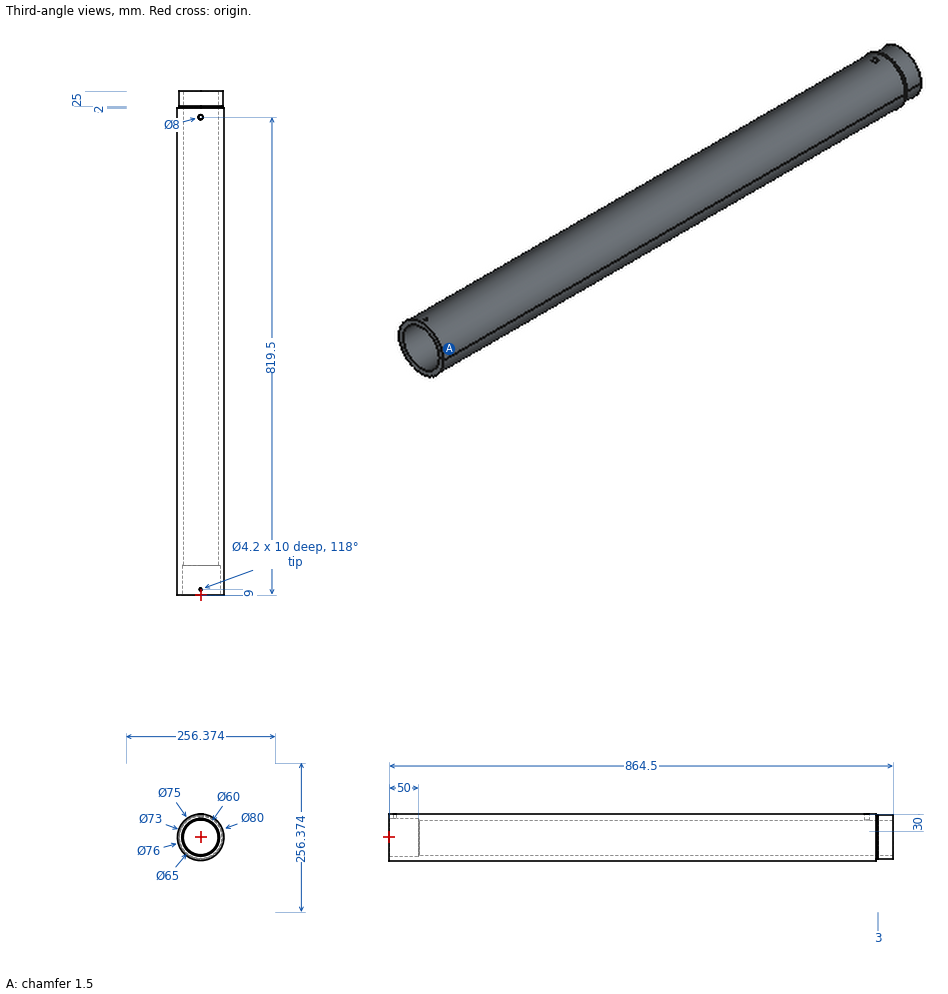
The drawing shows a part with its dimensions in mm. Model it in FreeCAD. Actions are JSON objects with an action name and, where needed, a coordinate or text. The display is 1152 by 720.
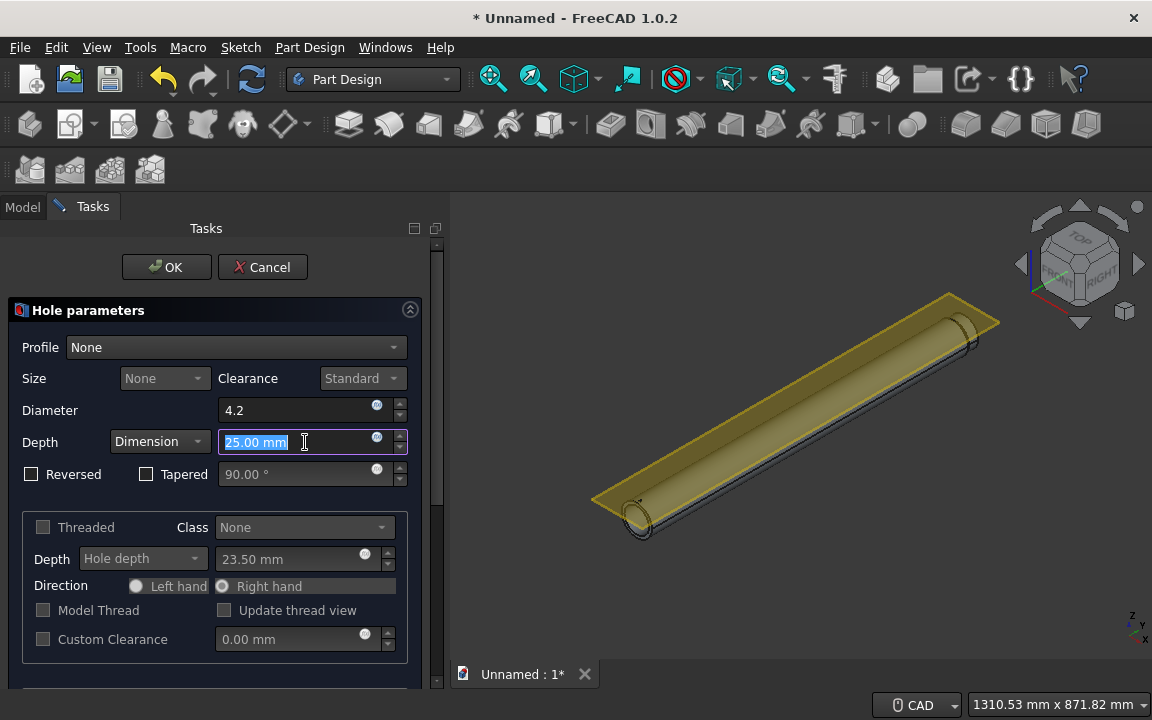
{"action": "type", "text": "10"}
{"action": "key", "text": "Tab"}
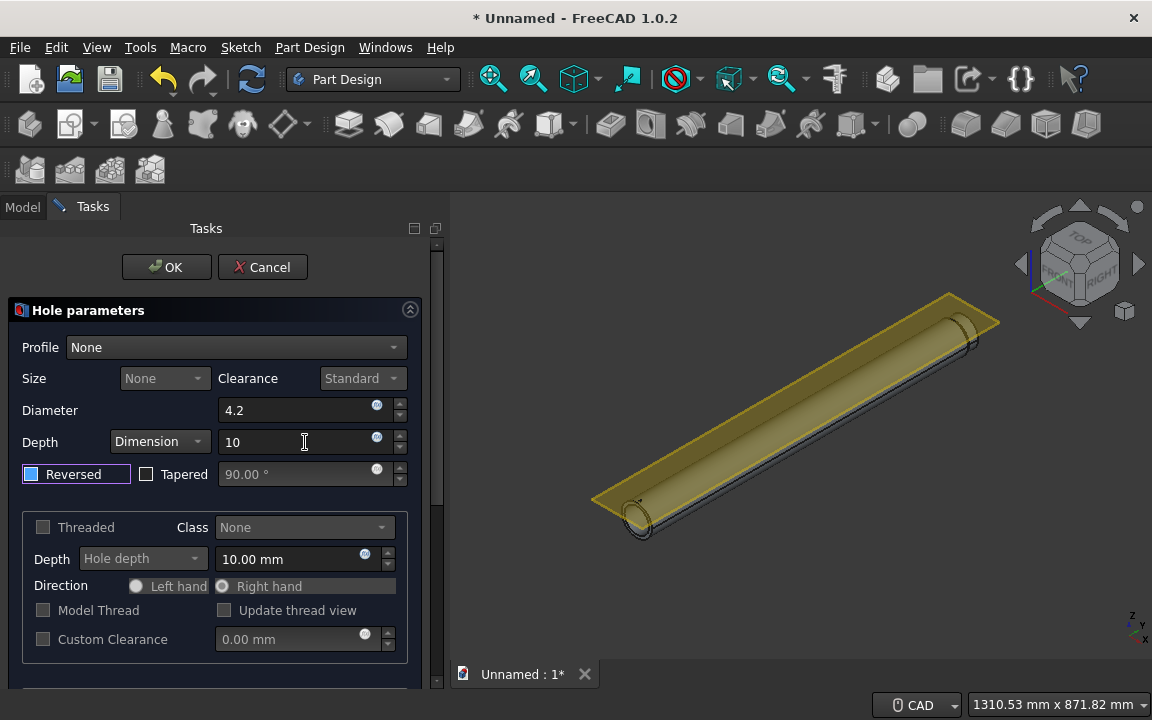
{"action": "left_click", "coordinate": [167, 267]}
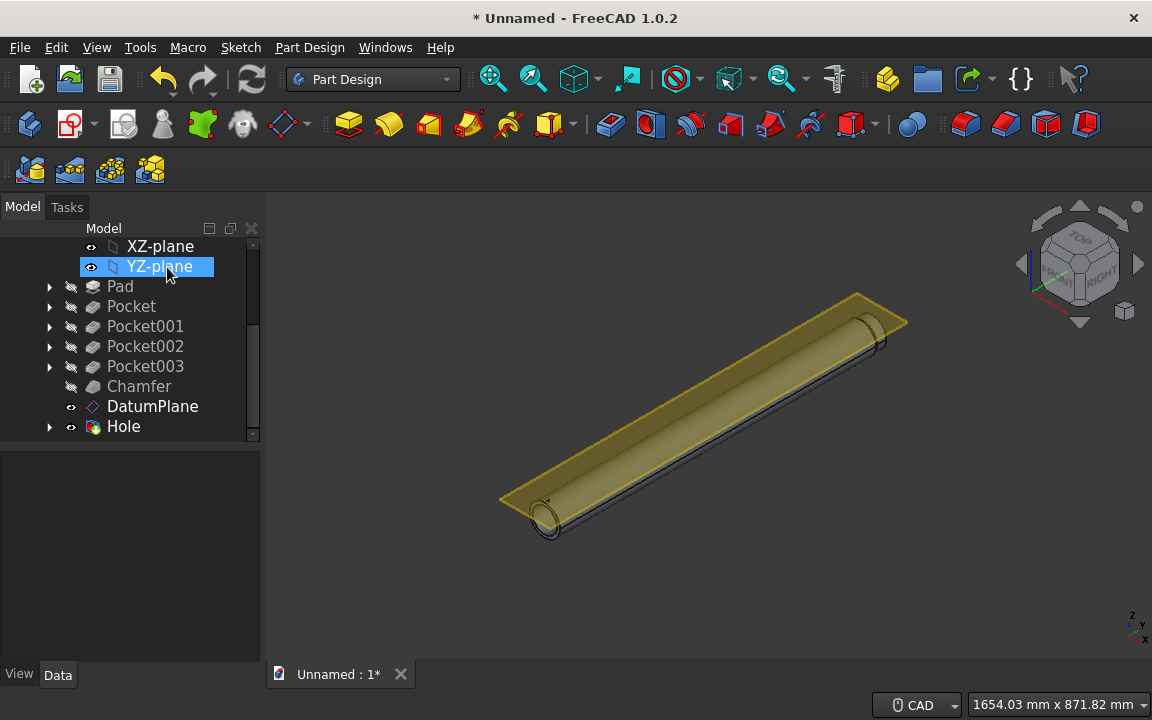
{"action": "left_click", "coordinate": [116, 407]}
{"action": "key", "text": "space"}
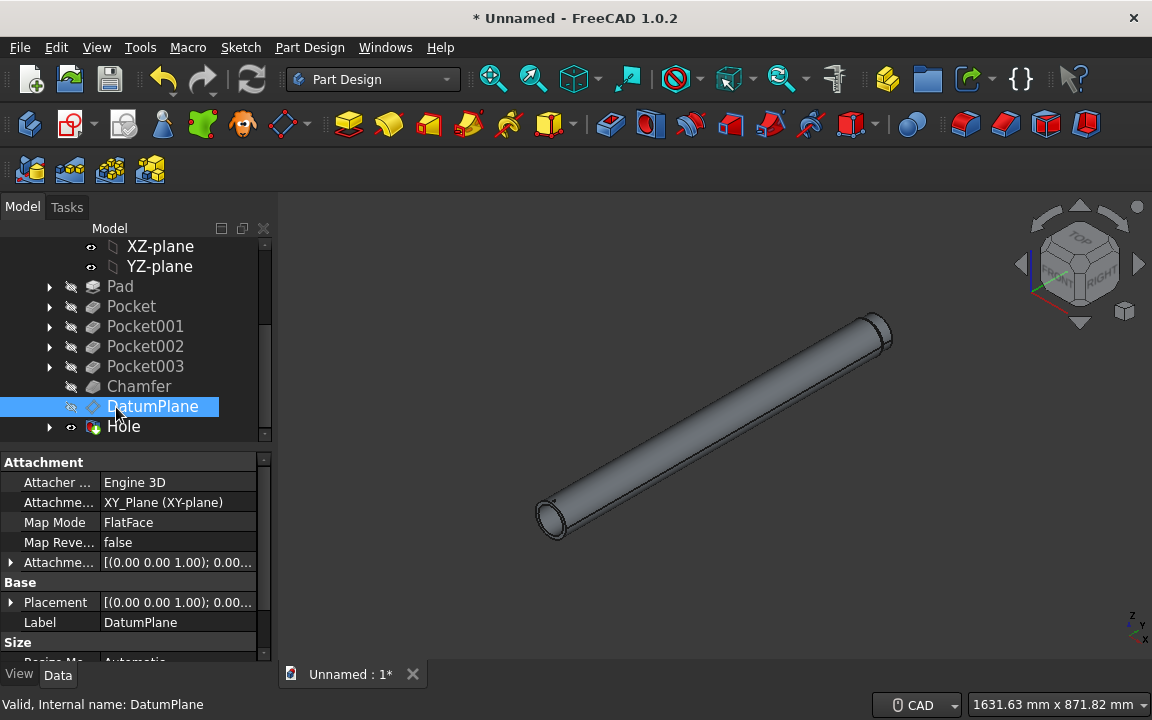
{"action": "scroll", "coordinate": [160, 342], "scroll_direction": "down", "scroll_amount": 3}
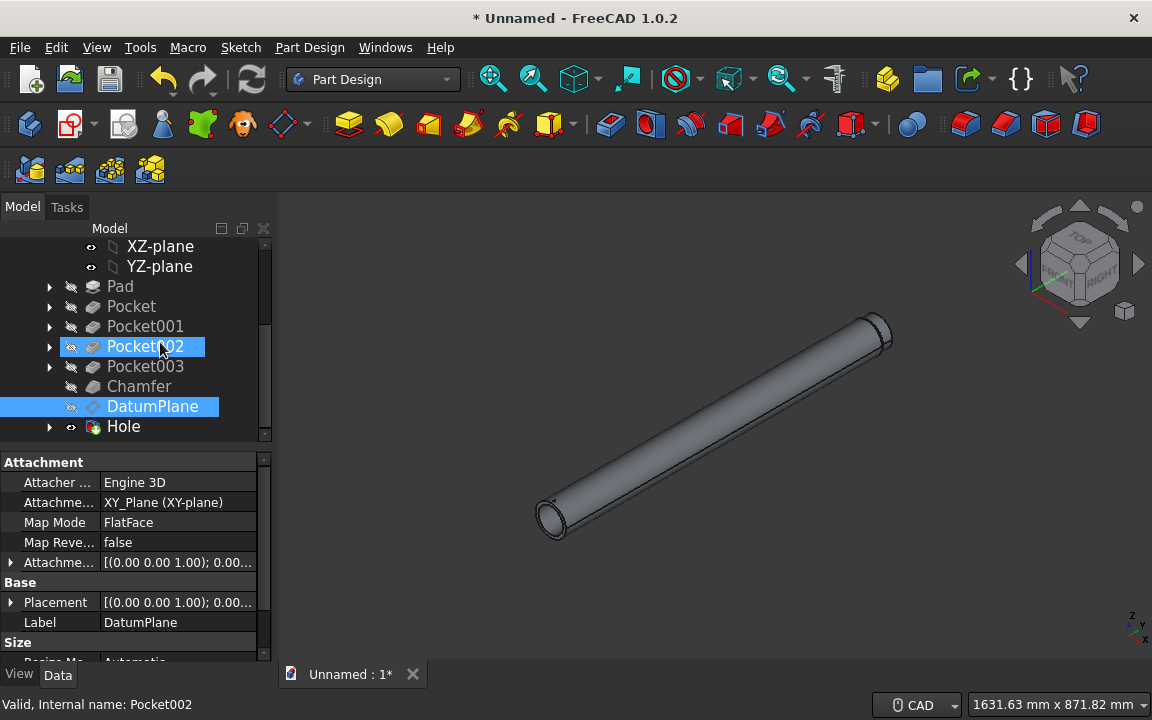
{"action": "scroll", "coordinate": [160, 342], "scroll_direction": "up", "scroll_amount": 15}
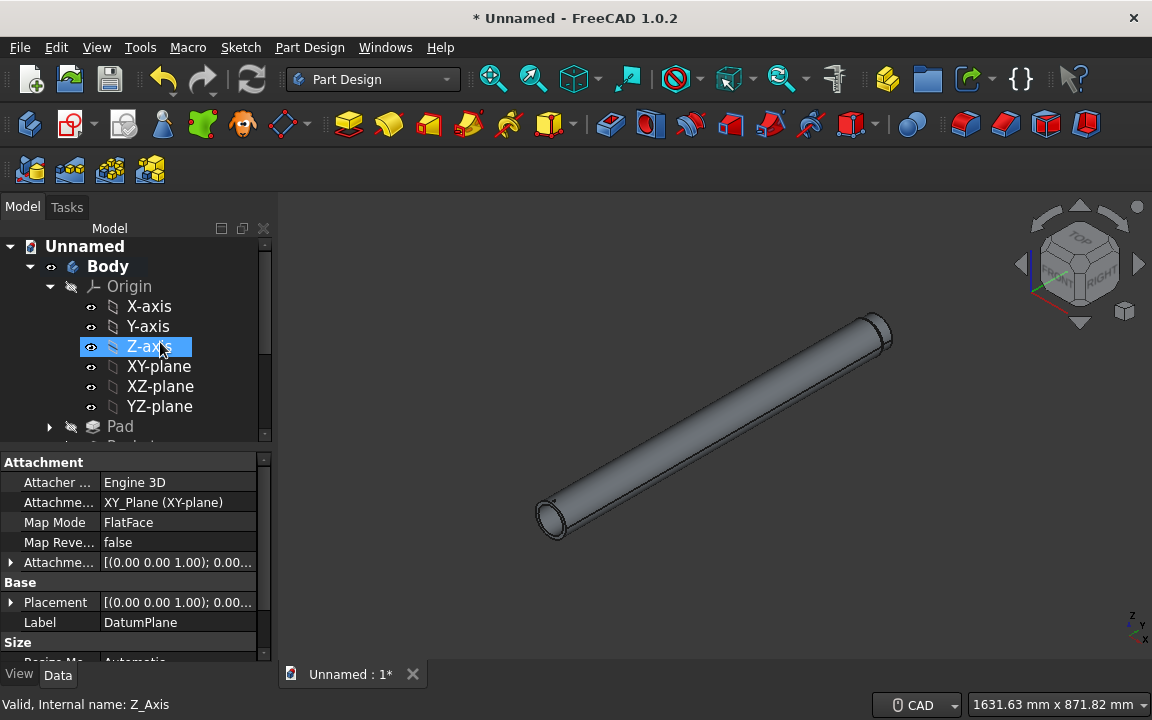
{"action": "left_click", "coordinate": [136, 367]}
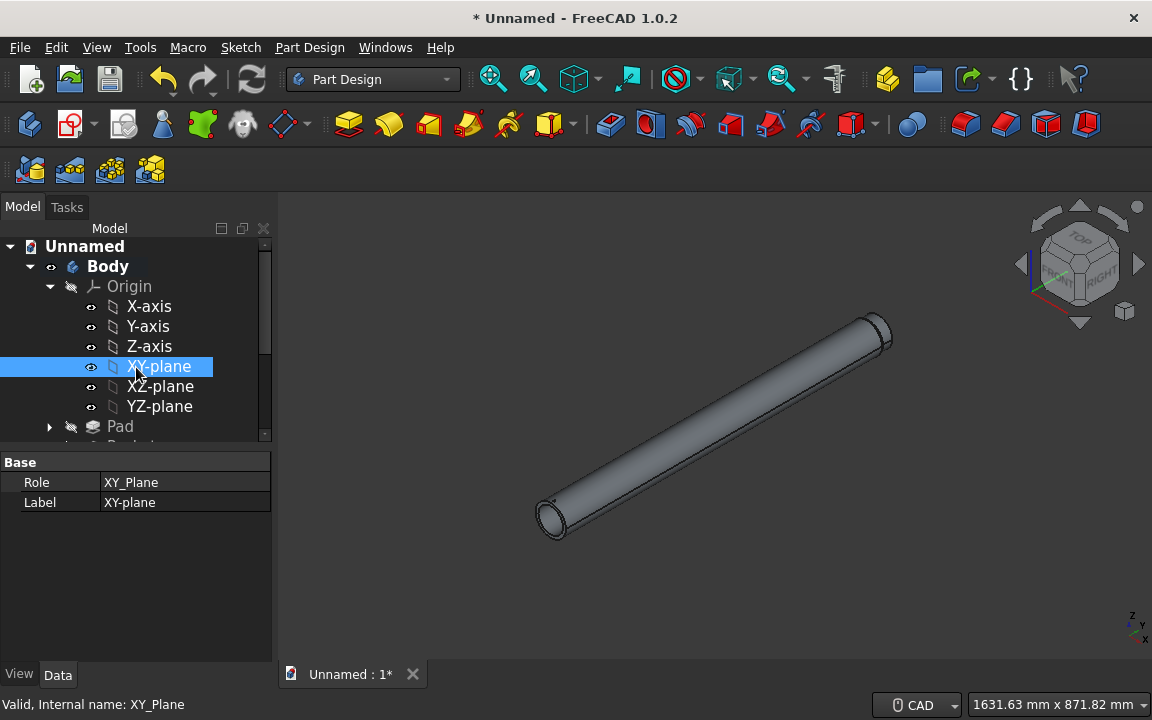
{"action": "left_click", "coordinate": [284, 124]}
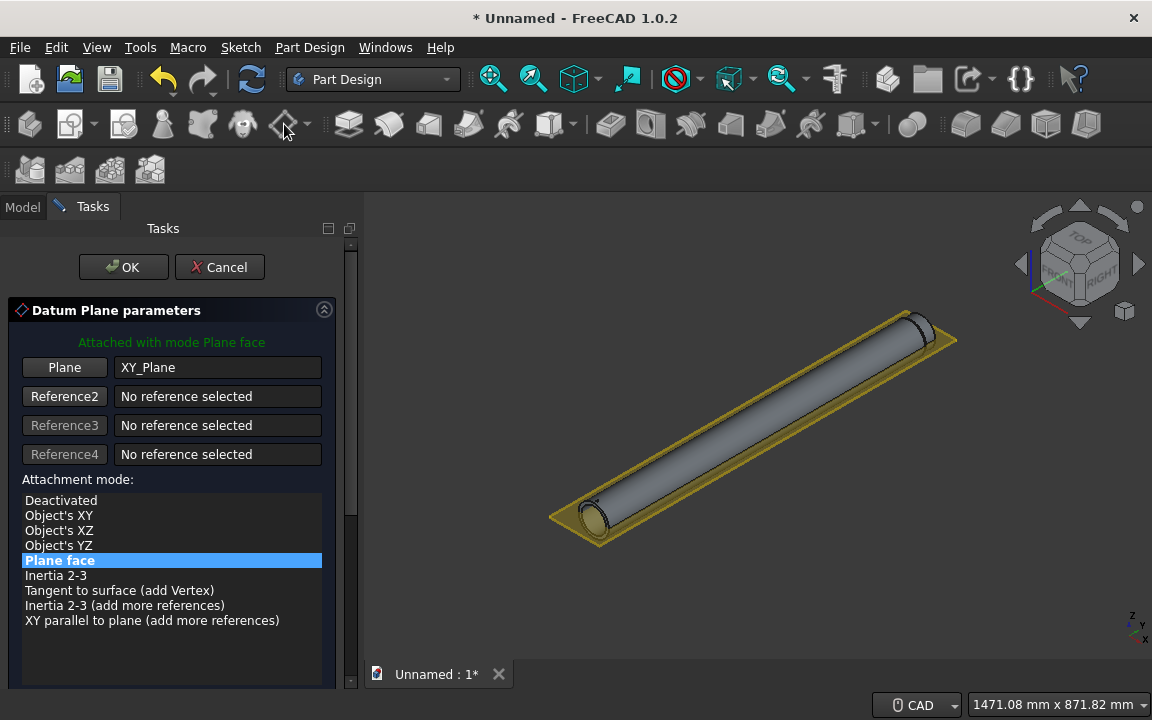
{"action": "scroll", "coordinate": [351, 463], "scroll_direction": "down", "scroll_amount": 3}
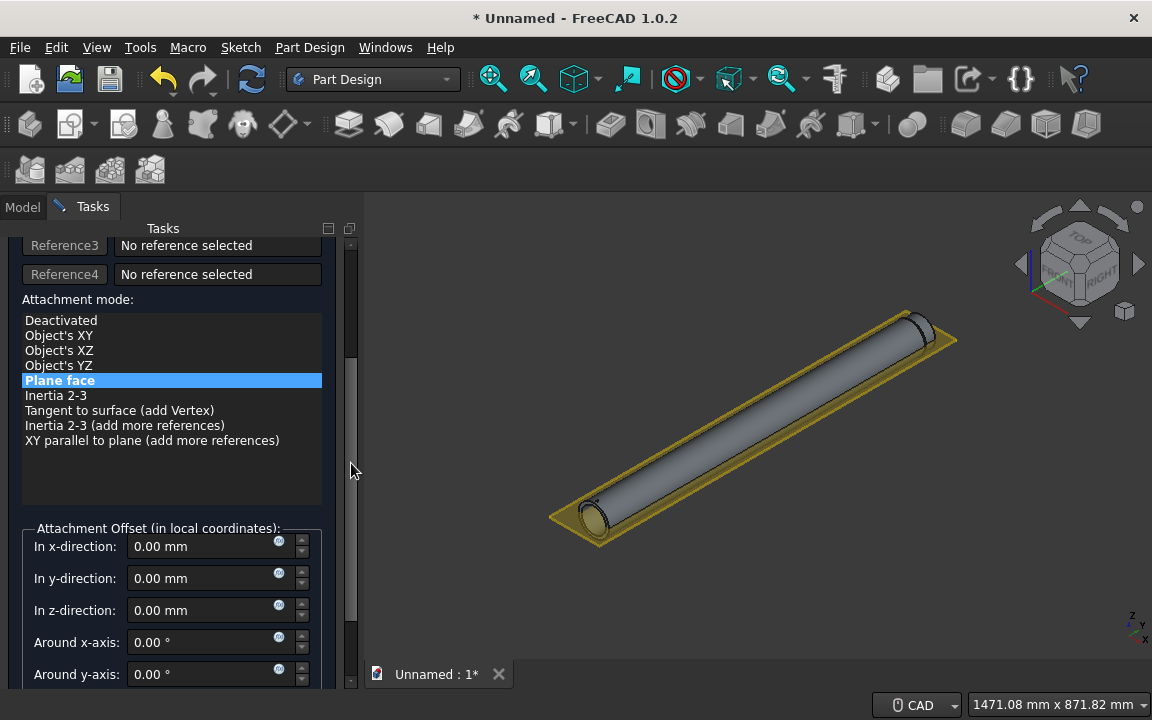
{"action": "triple_click", "coordinate": [210, 610]}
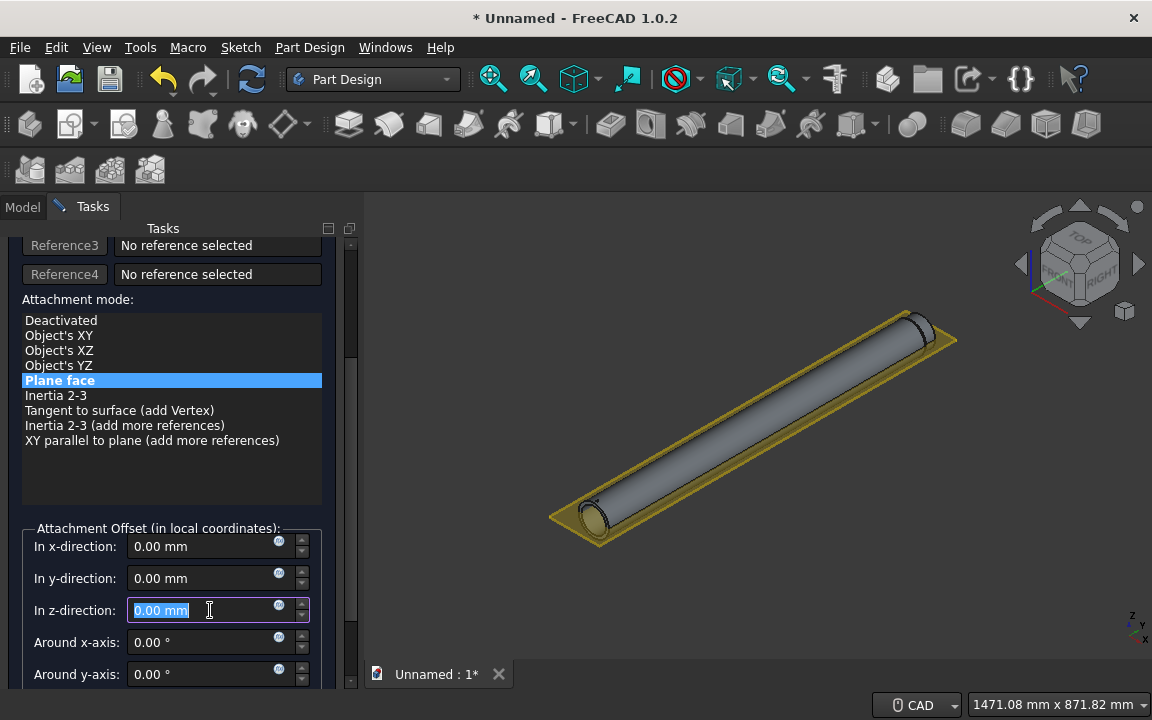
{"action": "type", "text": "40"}
{"action": "key", "text": "Tab"}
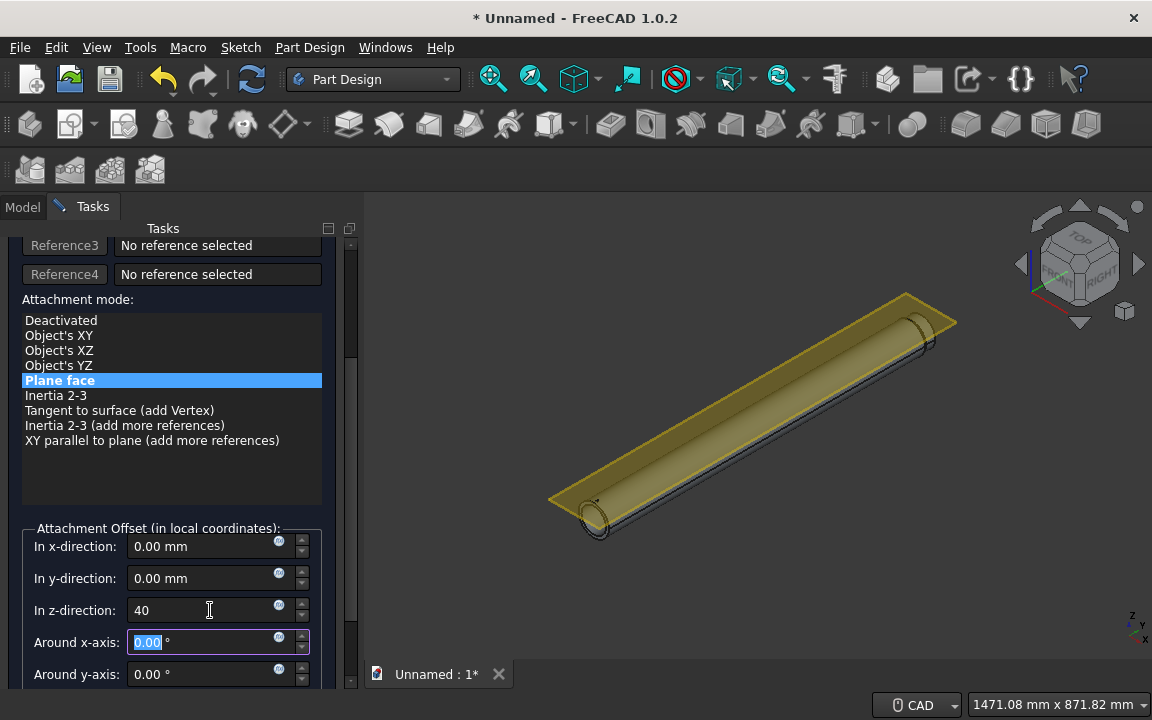
{"action": "scroll", "coordinate": [351, 463], "scroll_direction": "up", "scroll_amount": 4}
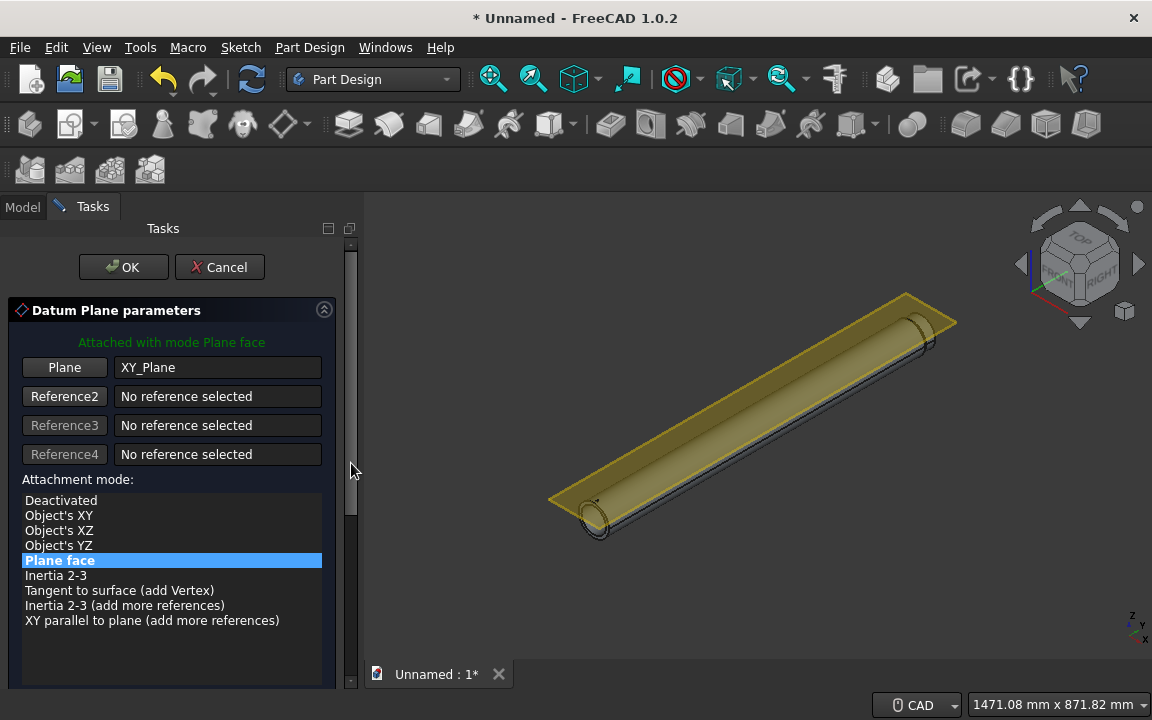
{"action": "left_click", "coordinate": [124, 267]}